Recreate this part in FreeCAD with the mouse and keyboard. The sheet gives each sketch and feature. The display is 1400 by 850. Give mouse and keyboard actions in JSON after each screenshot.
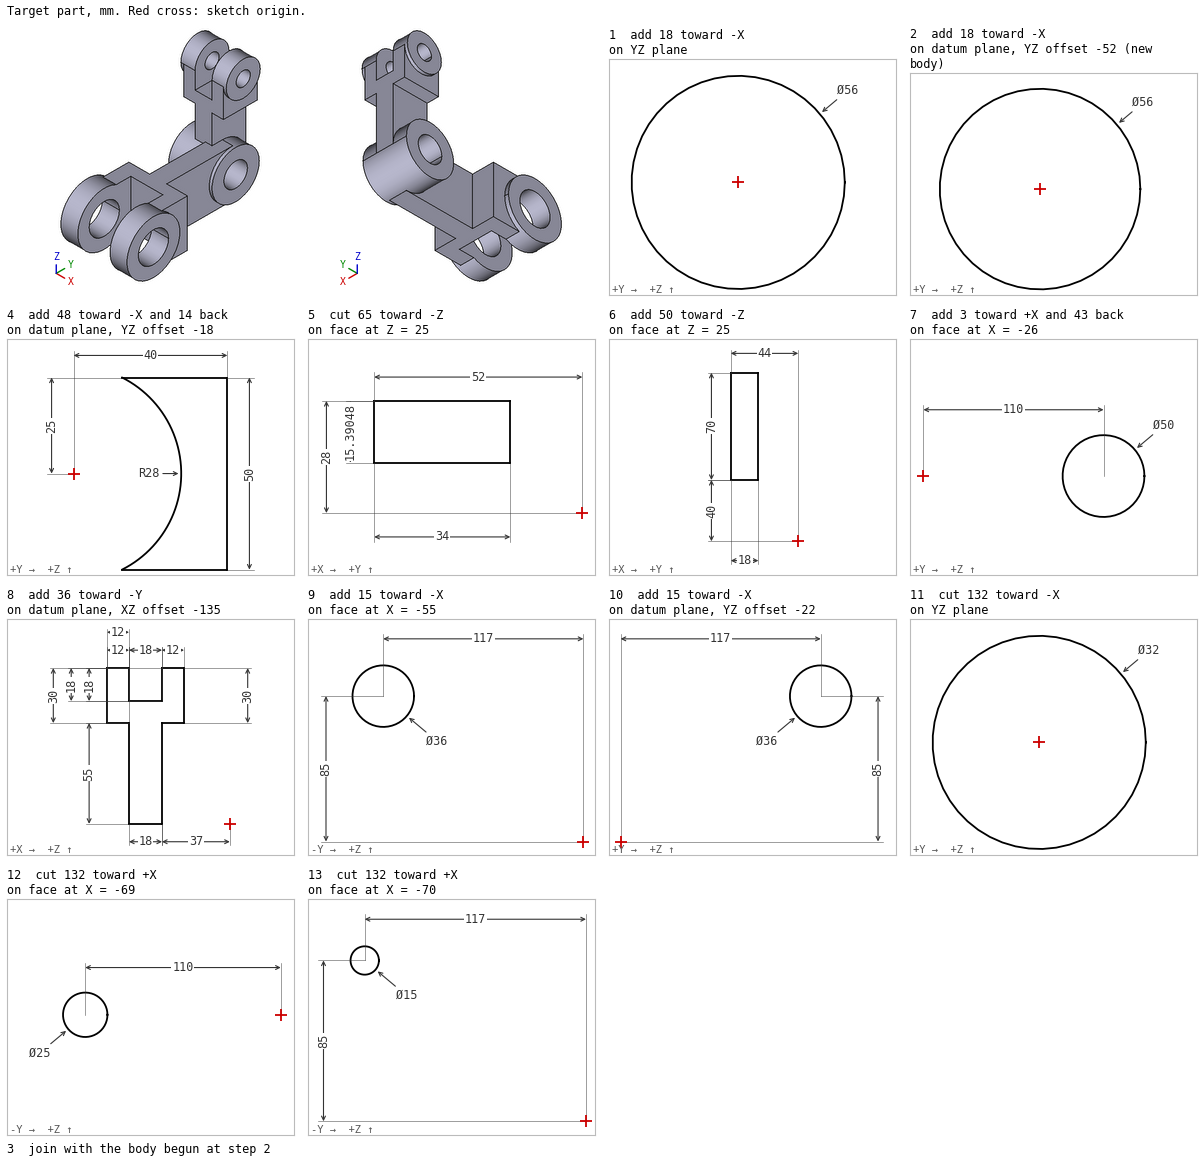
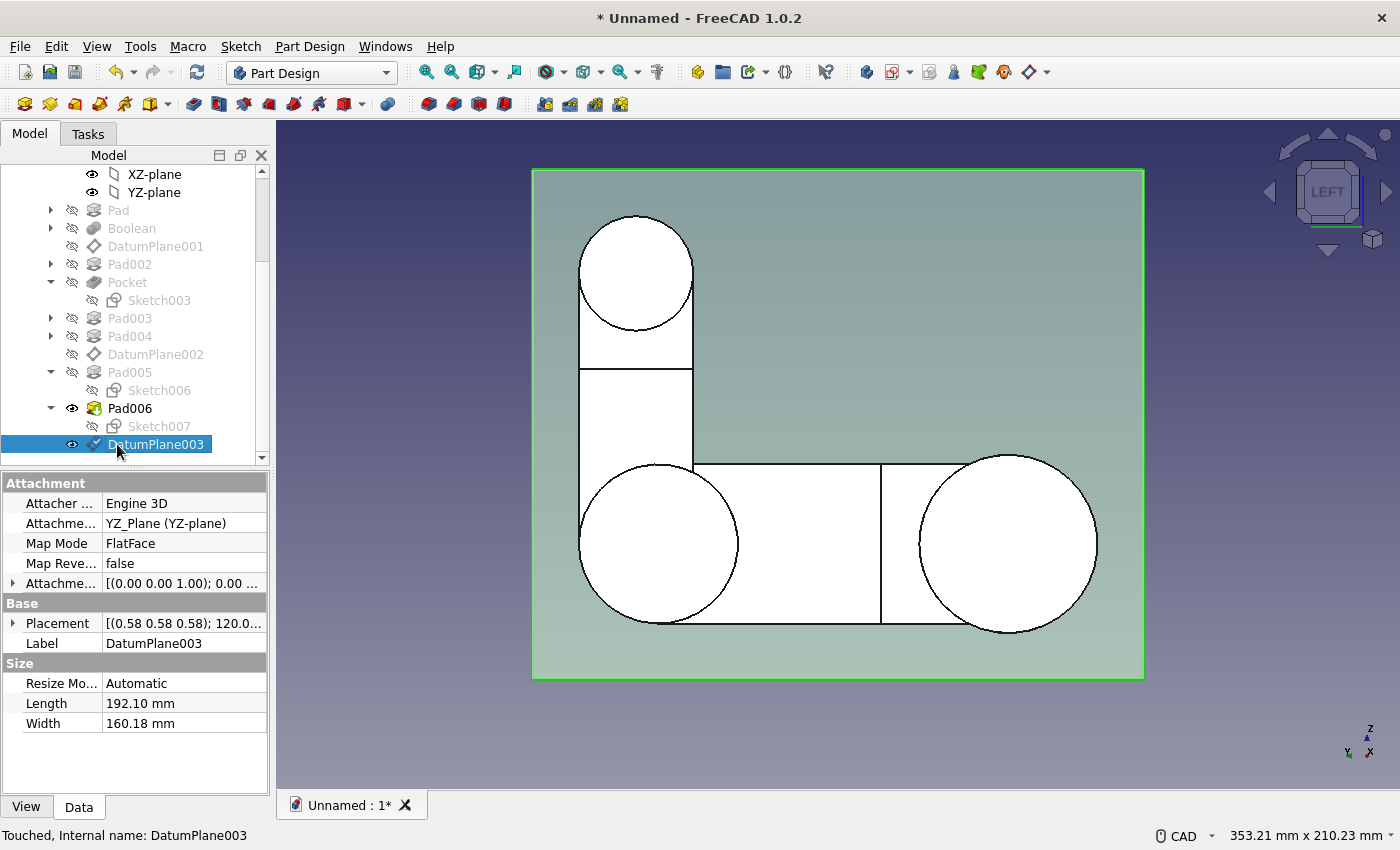
{"action": "left_click", "coordinate": [892, 72]}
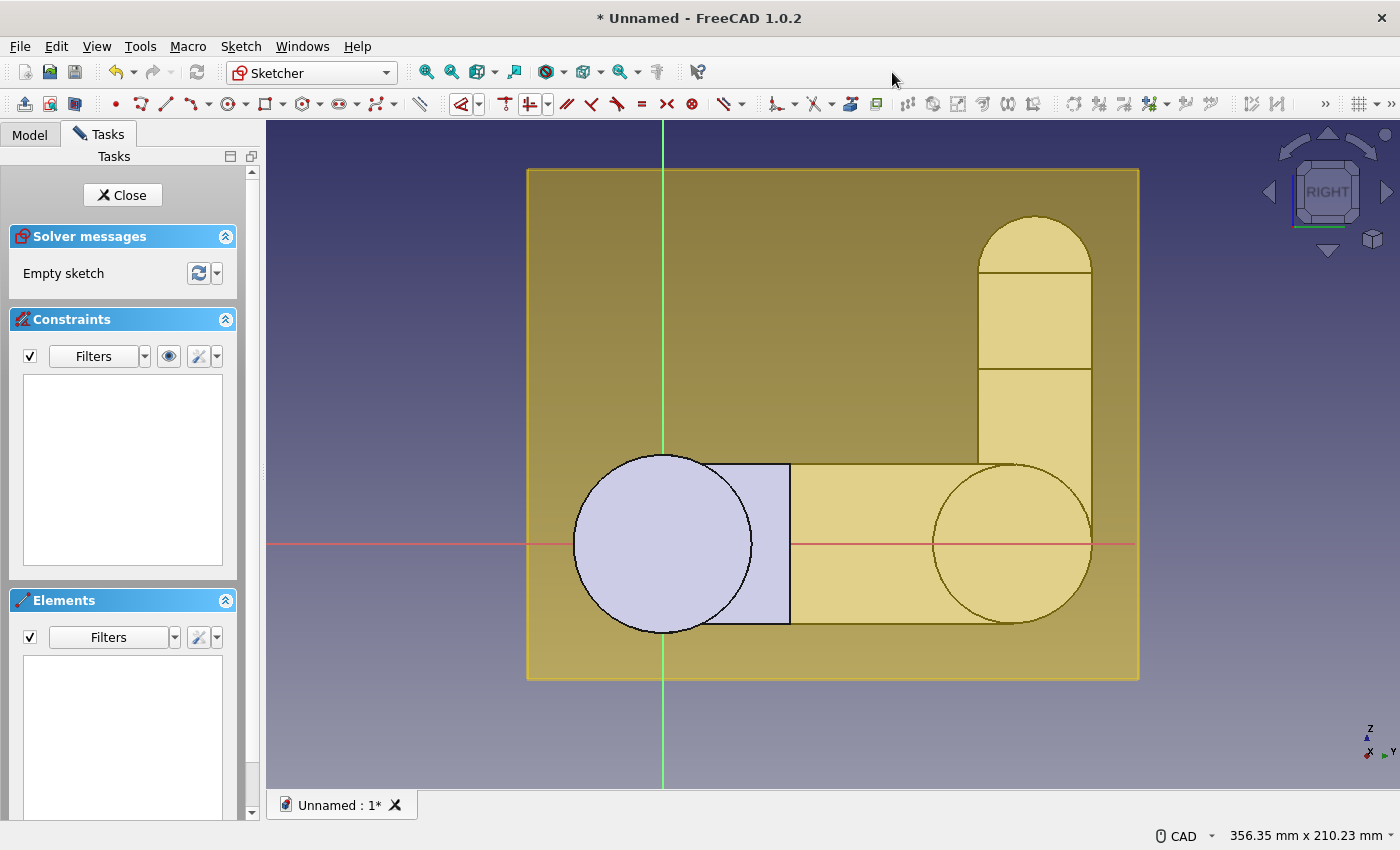
{"action": "key", "text": "q s"}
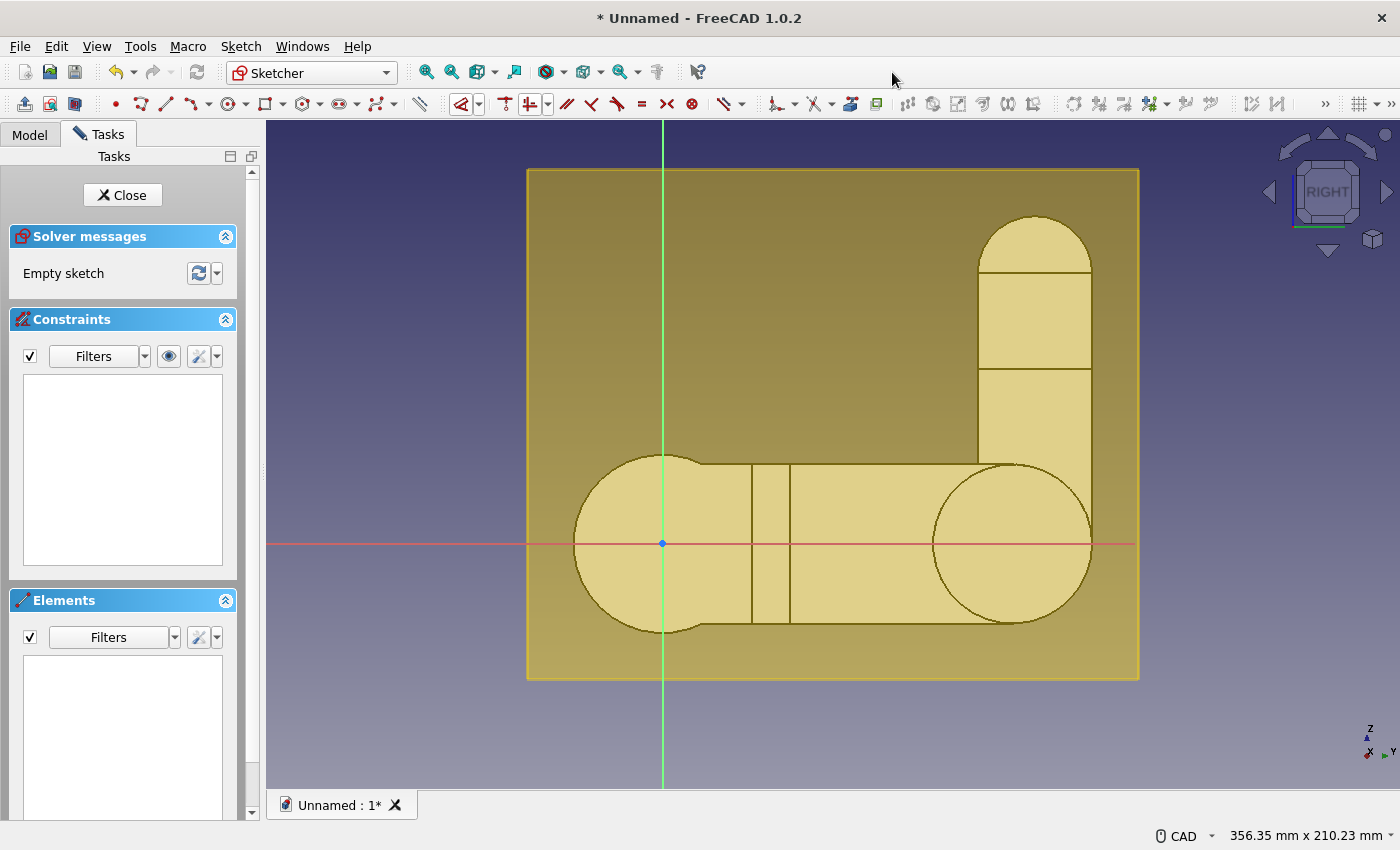
{"action": "scroll", "coordinate": [1123, 214], "scroll_direction": "up", "scroll_amount": 7}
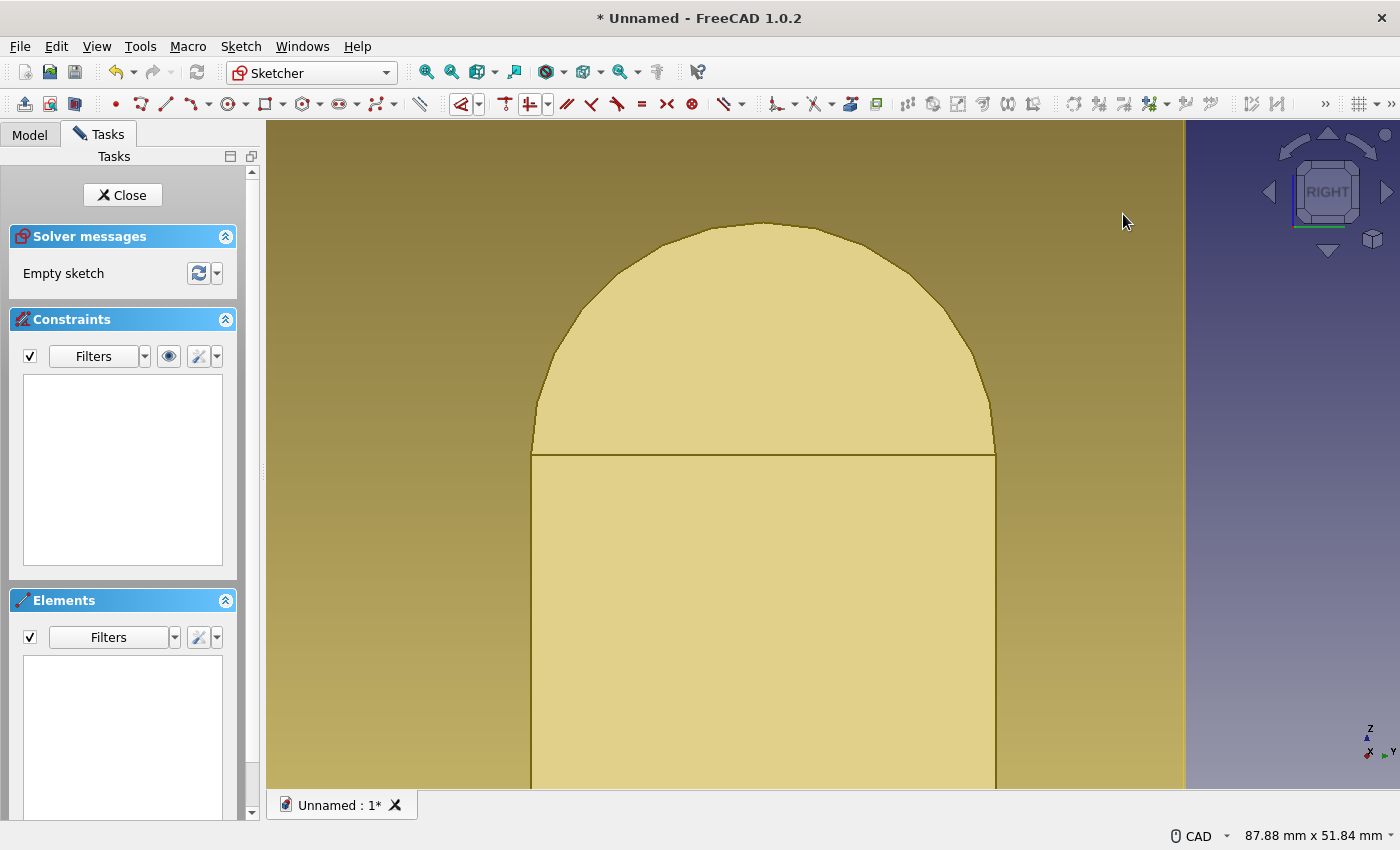
{"action": "left_click", "coordinate": [228, 104]}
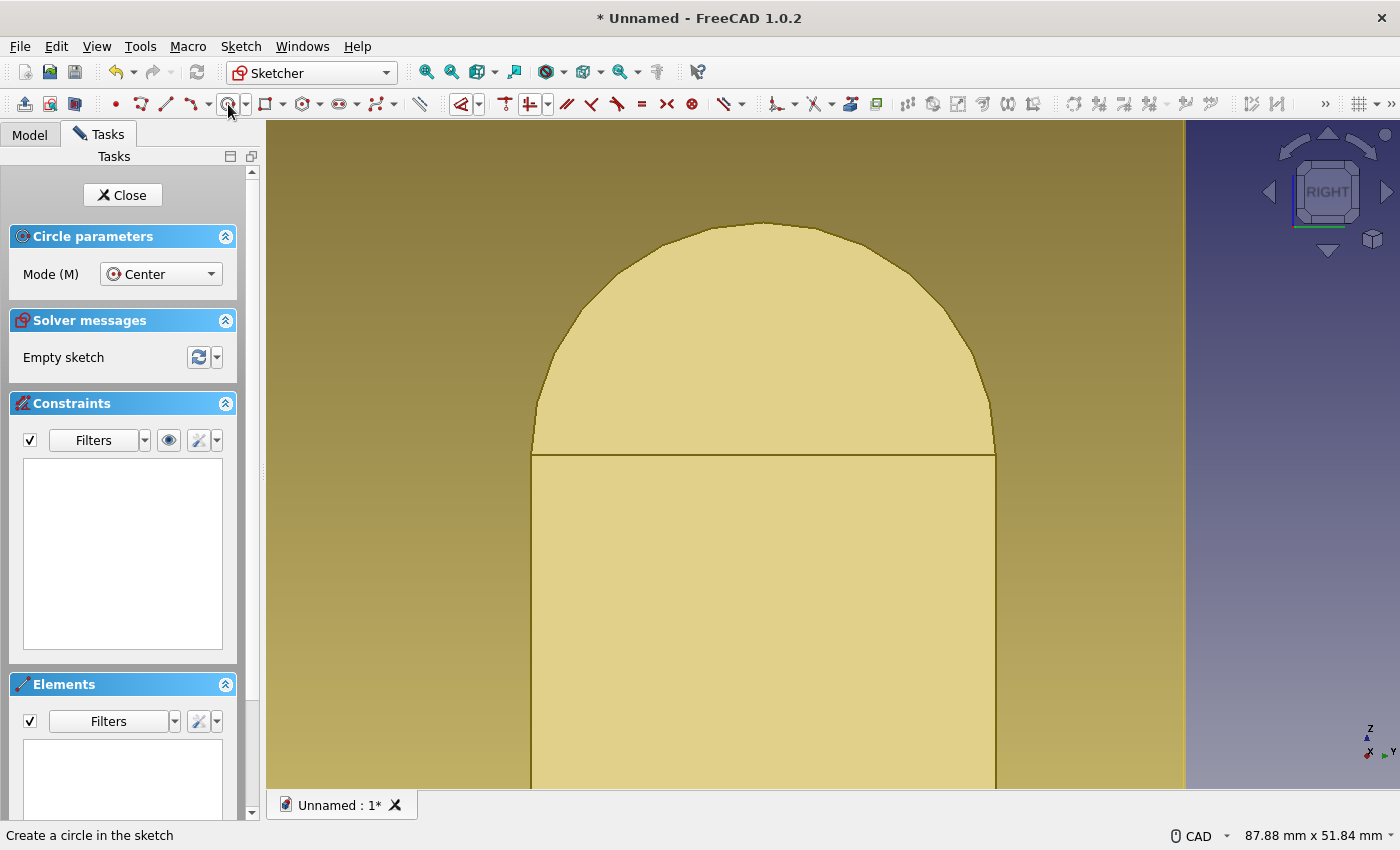
{"action": "left_click", "coordinate": [763, 455]}
{"action": "left_click", "coordinate": [928, 290]}
{"action": "key", "text": "Escape"}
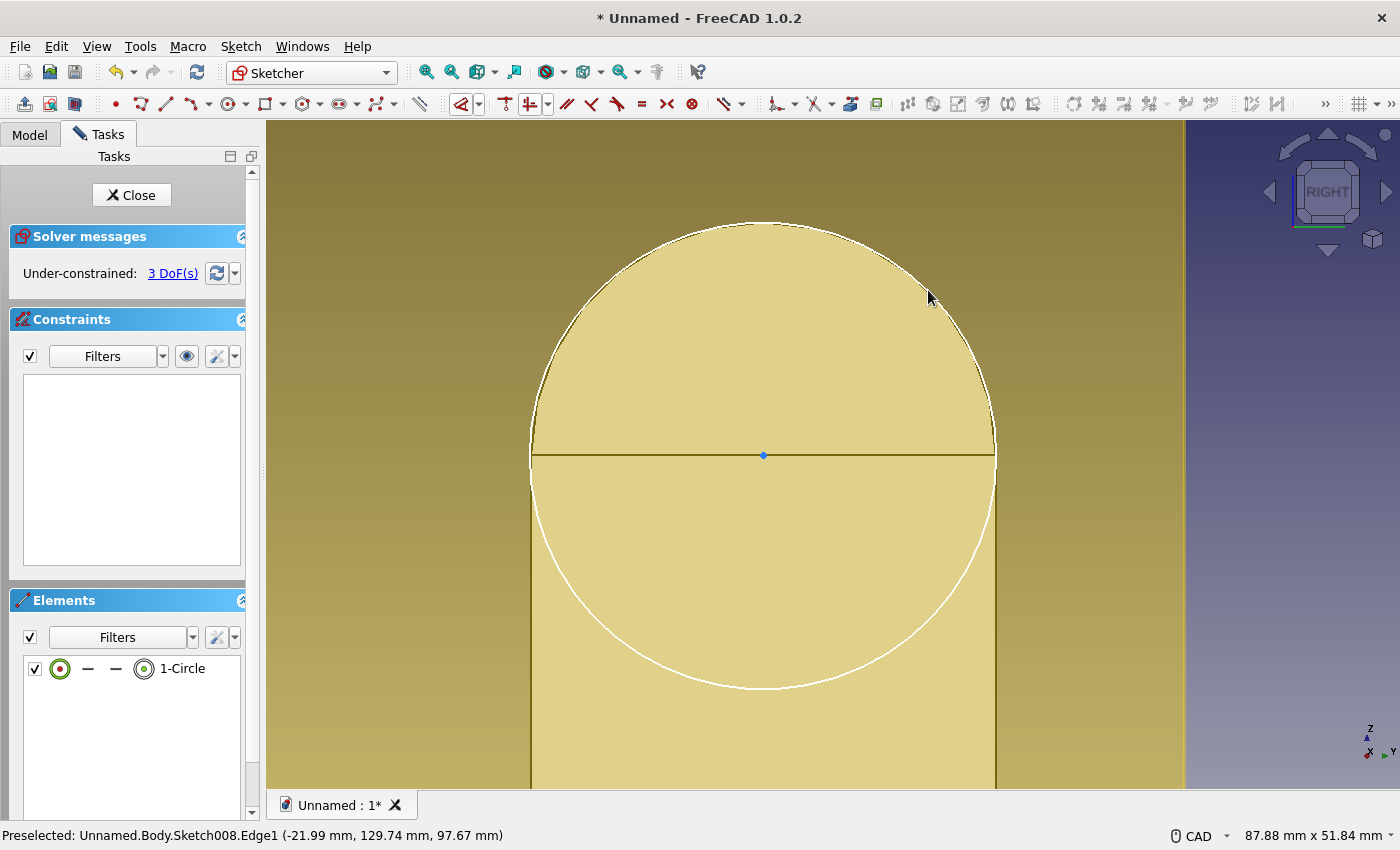
{"action": "left_click", "coordinate": [927, 290]}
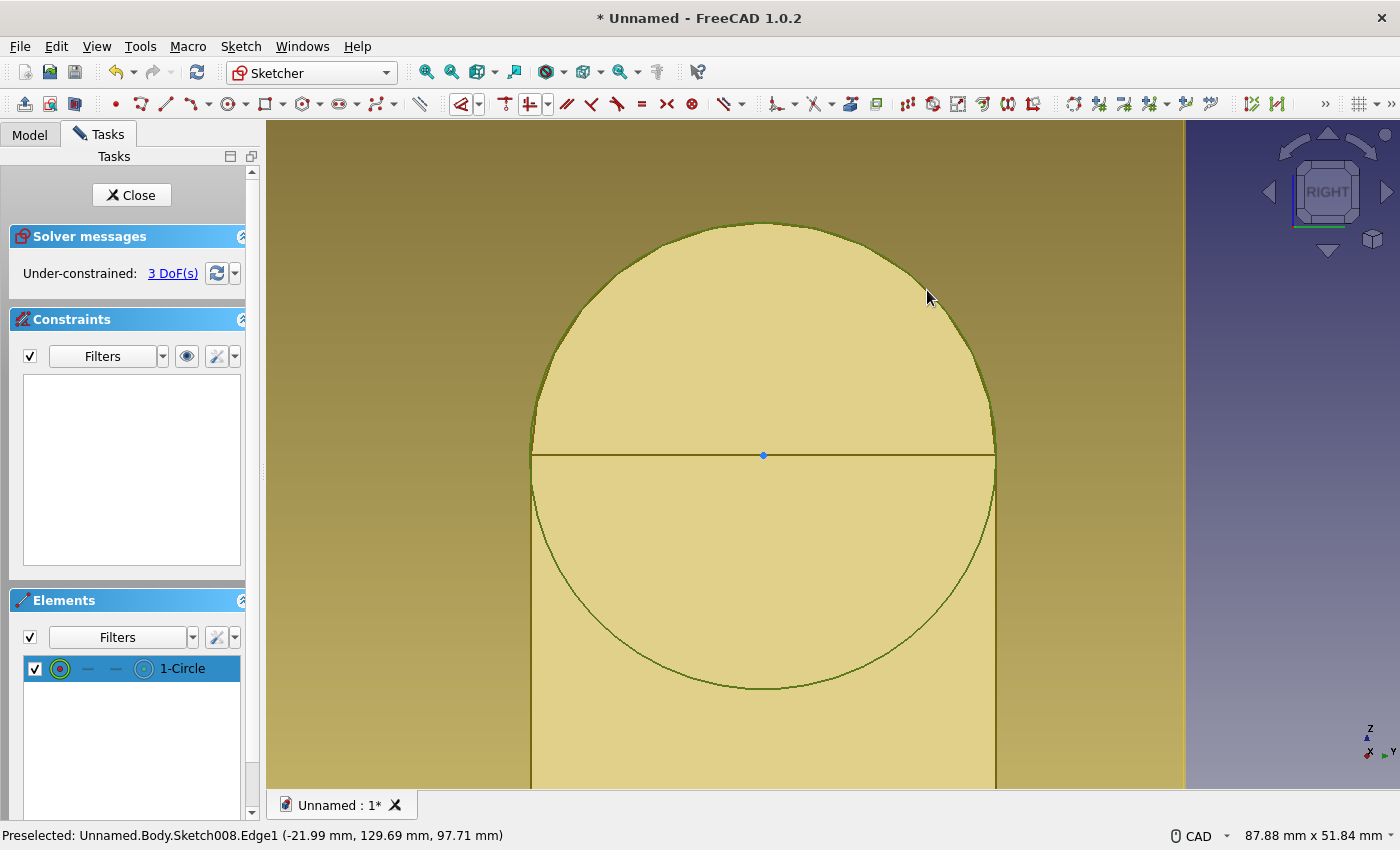
{"action": "left_click", "coordinate": [478, 104]}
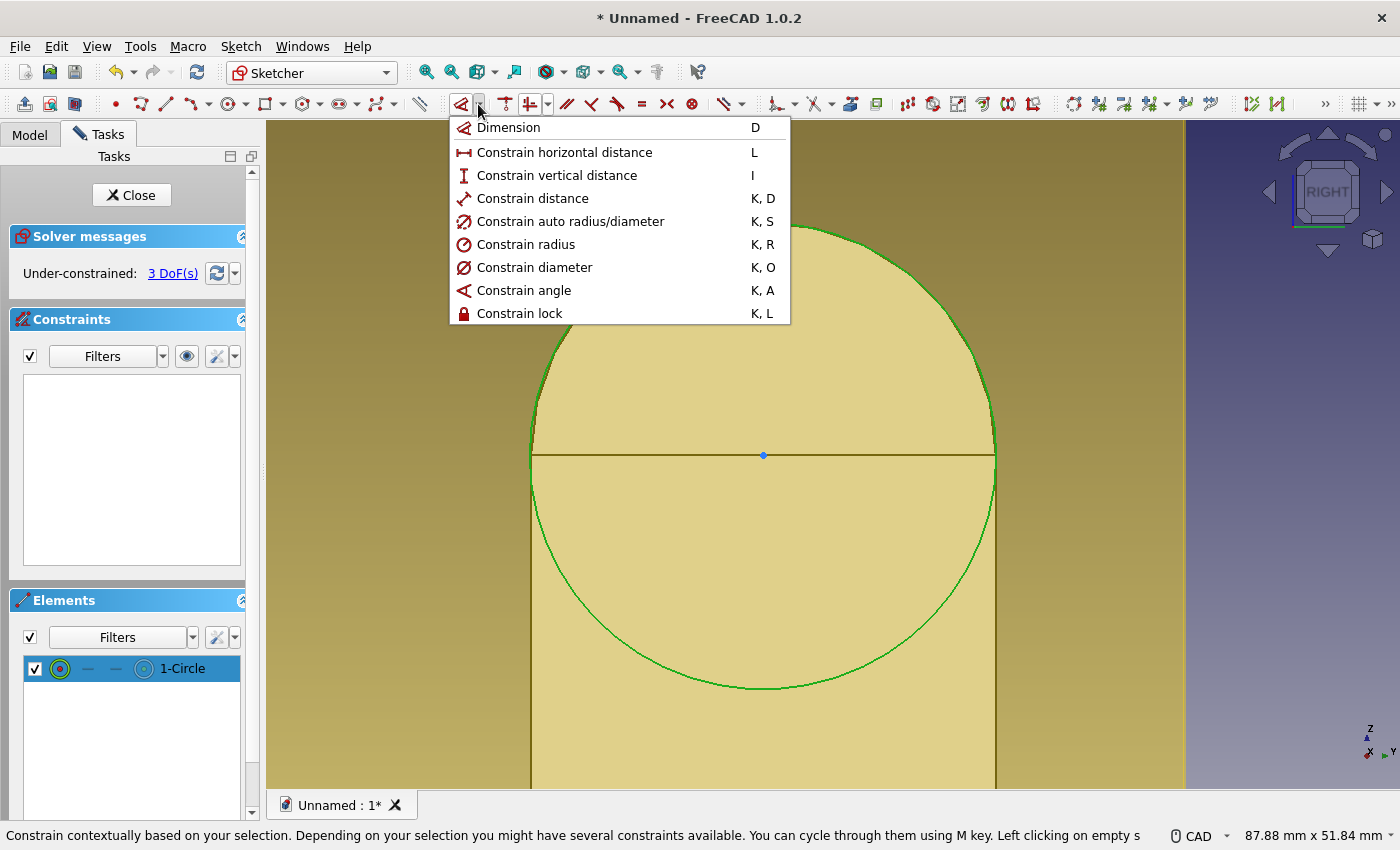
{"action": "left_click", "coordinate": [620, 268]}